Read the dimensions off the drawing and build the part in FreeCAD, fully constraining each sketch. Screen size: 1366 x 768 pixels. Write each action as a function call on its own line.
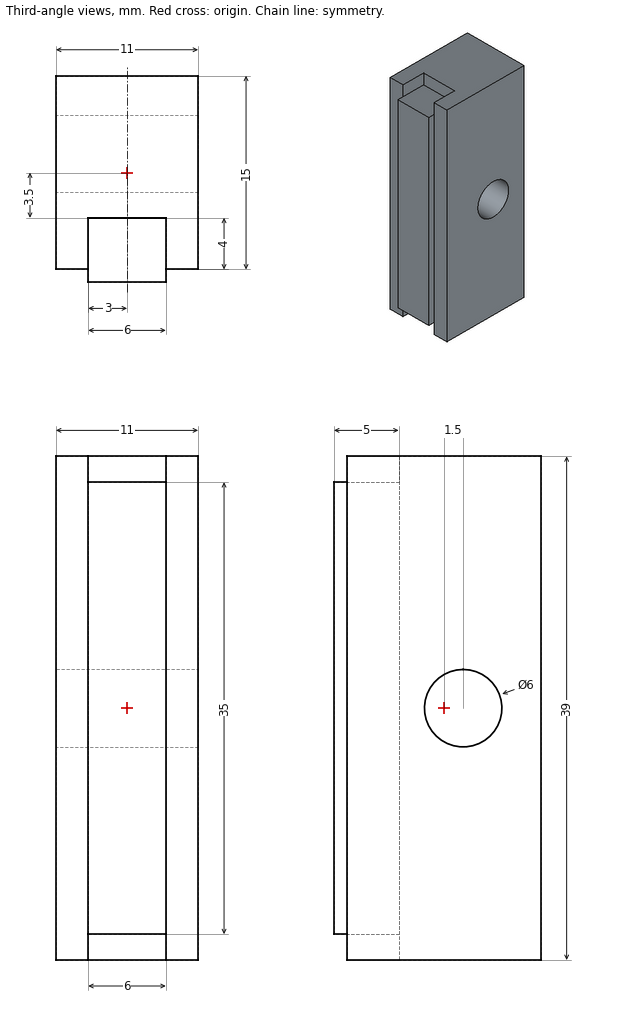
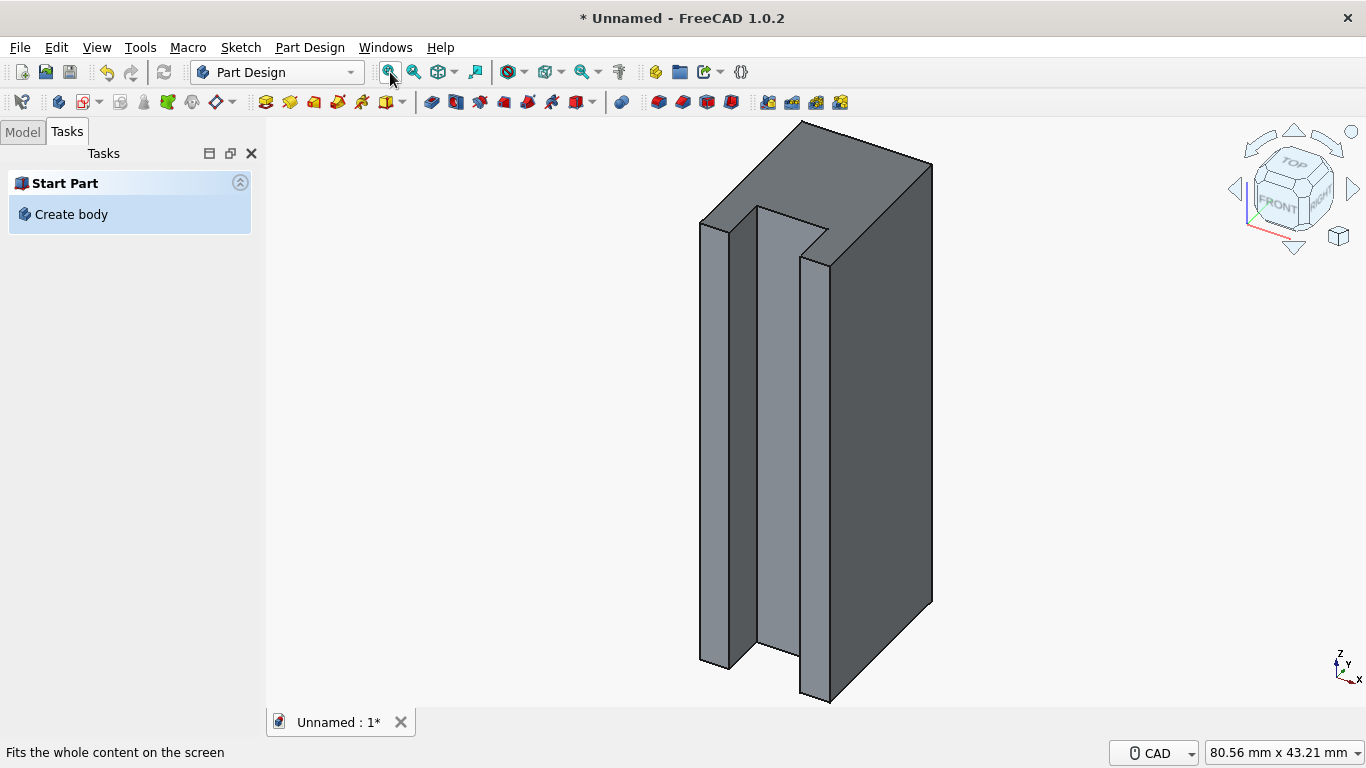
key(6)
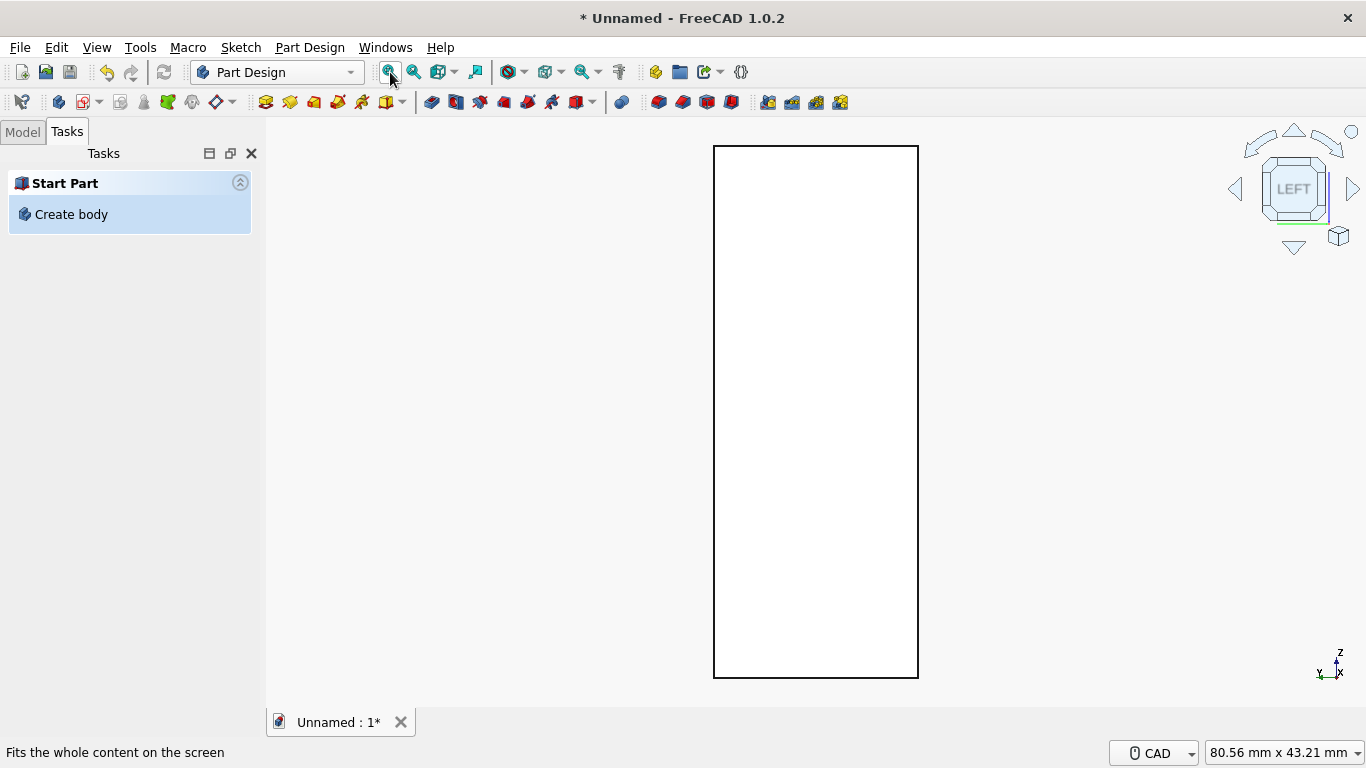
click(816, 259)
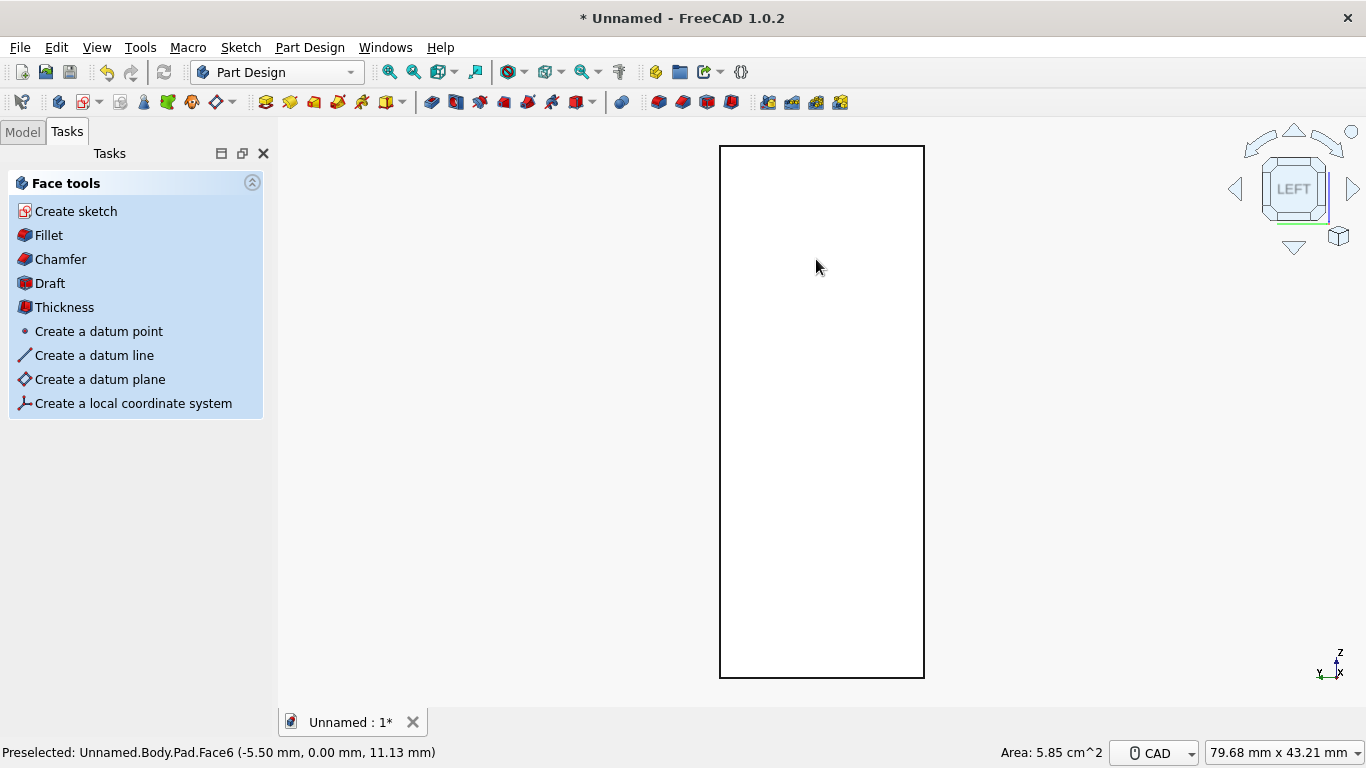
click(84, 102)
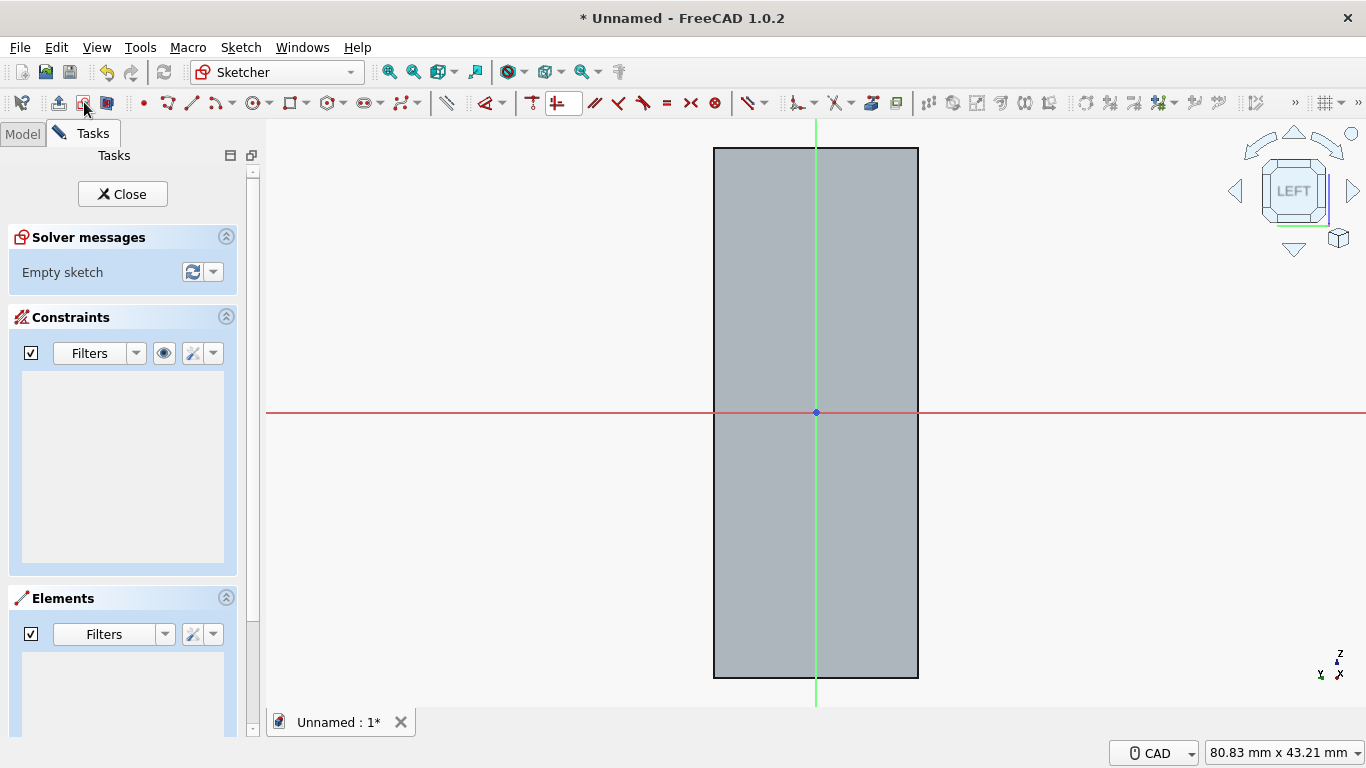
scroll(808, 413, up, 8)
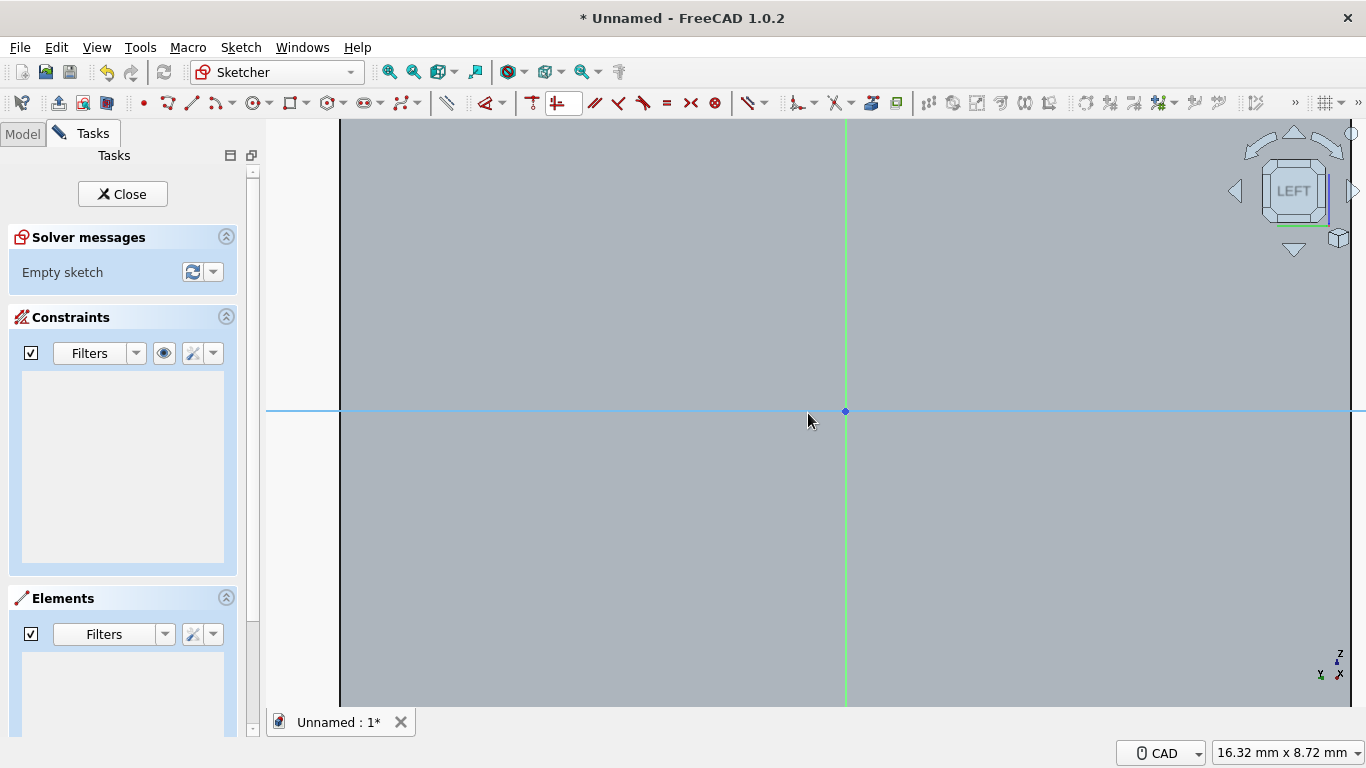
click(254, 104)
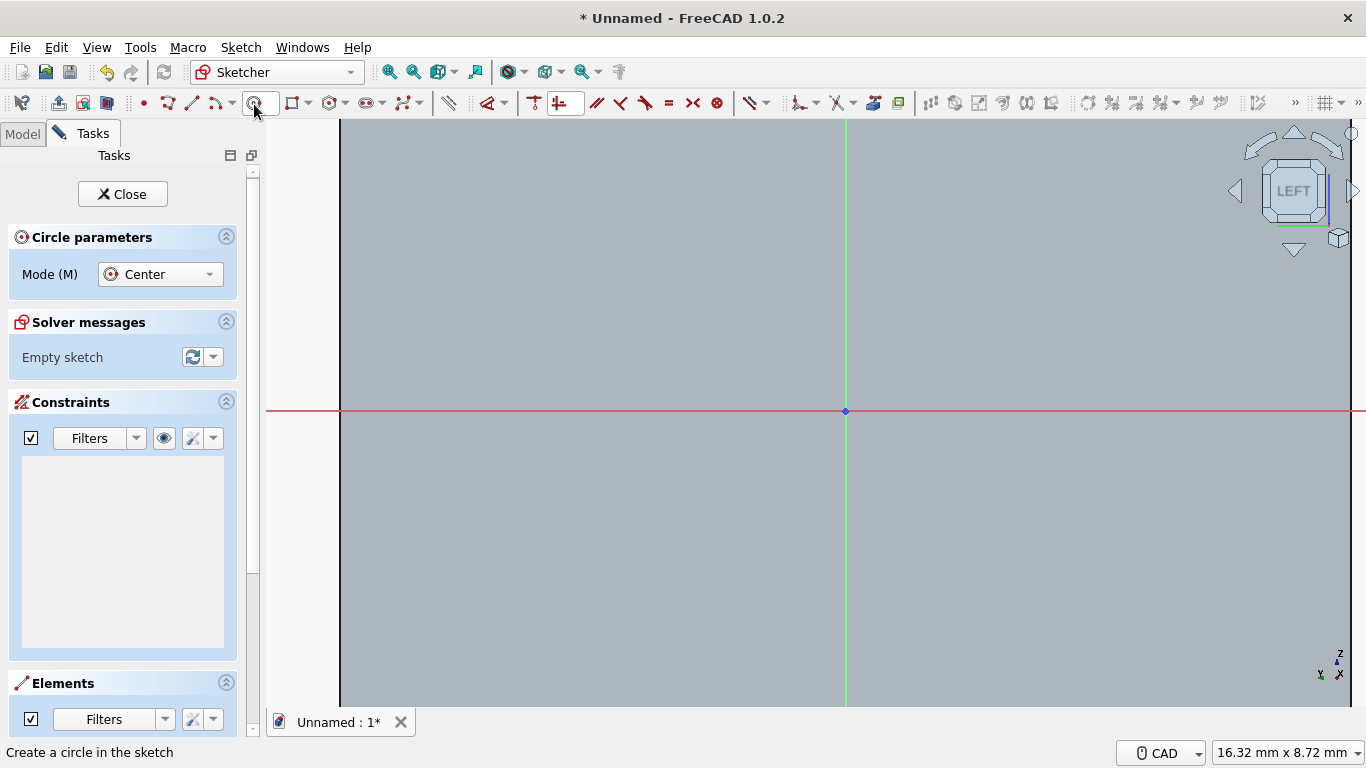
click(745, 411)
click(888, 268)
key(Escape)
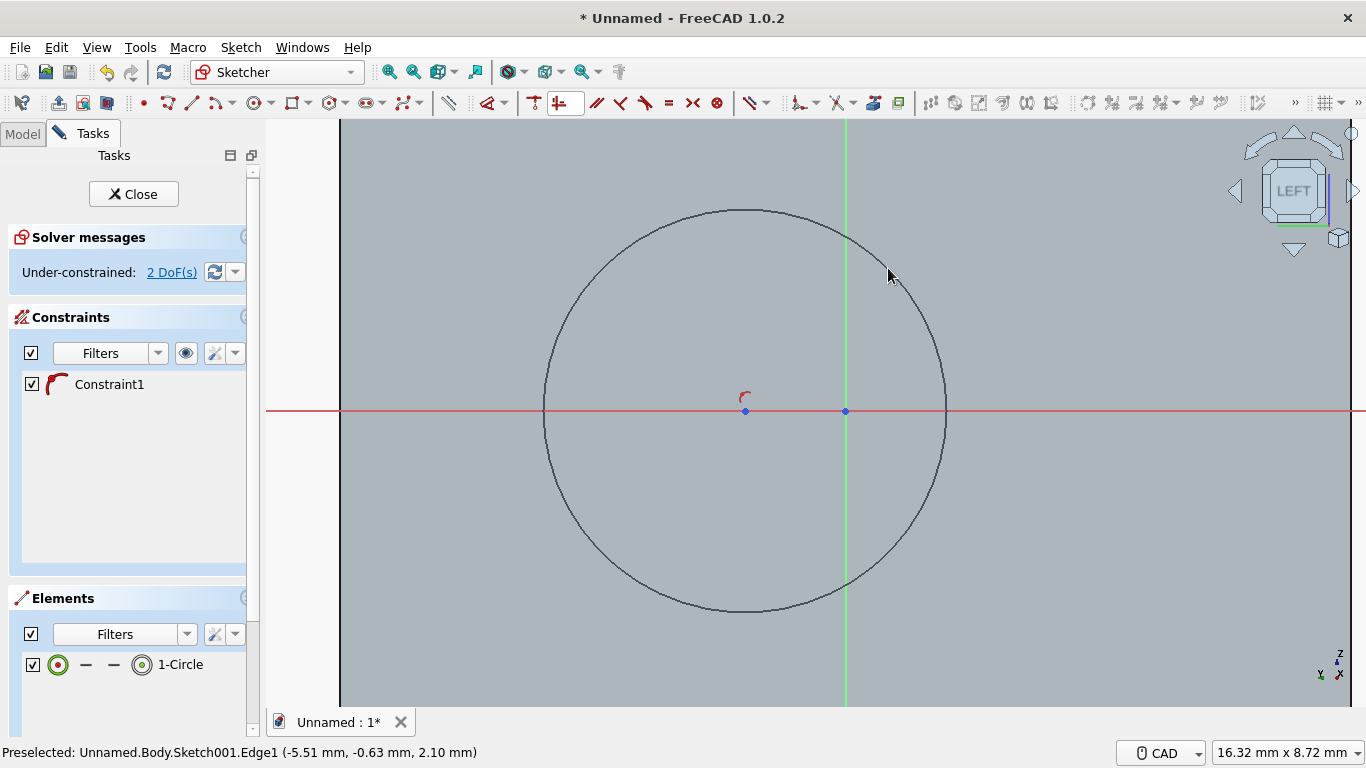
click(488, 104)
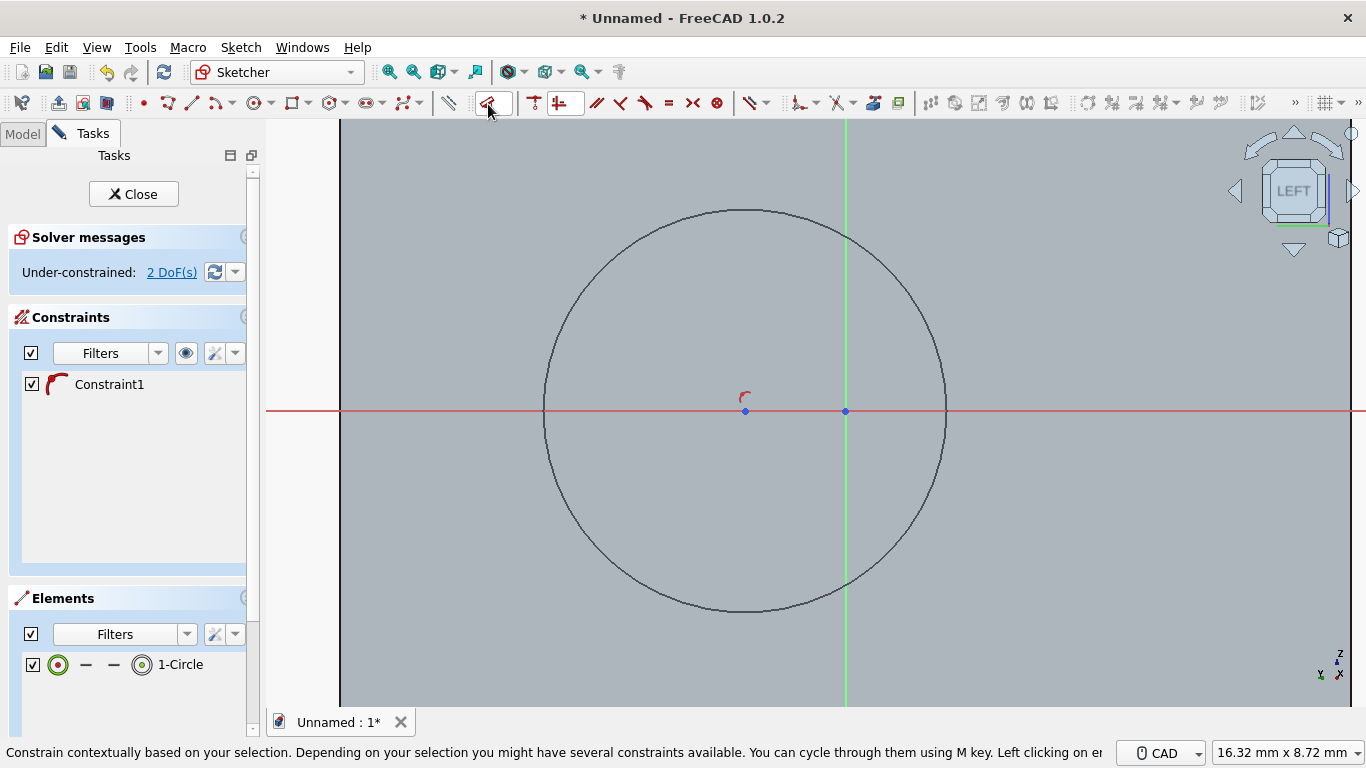
click(887, 268)
click(910, 245)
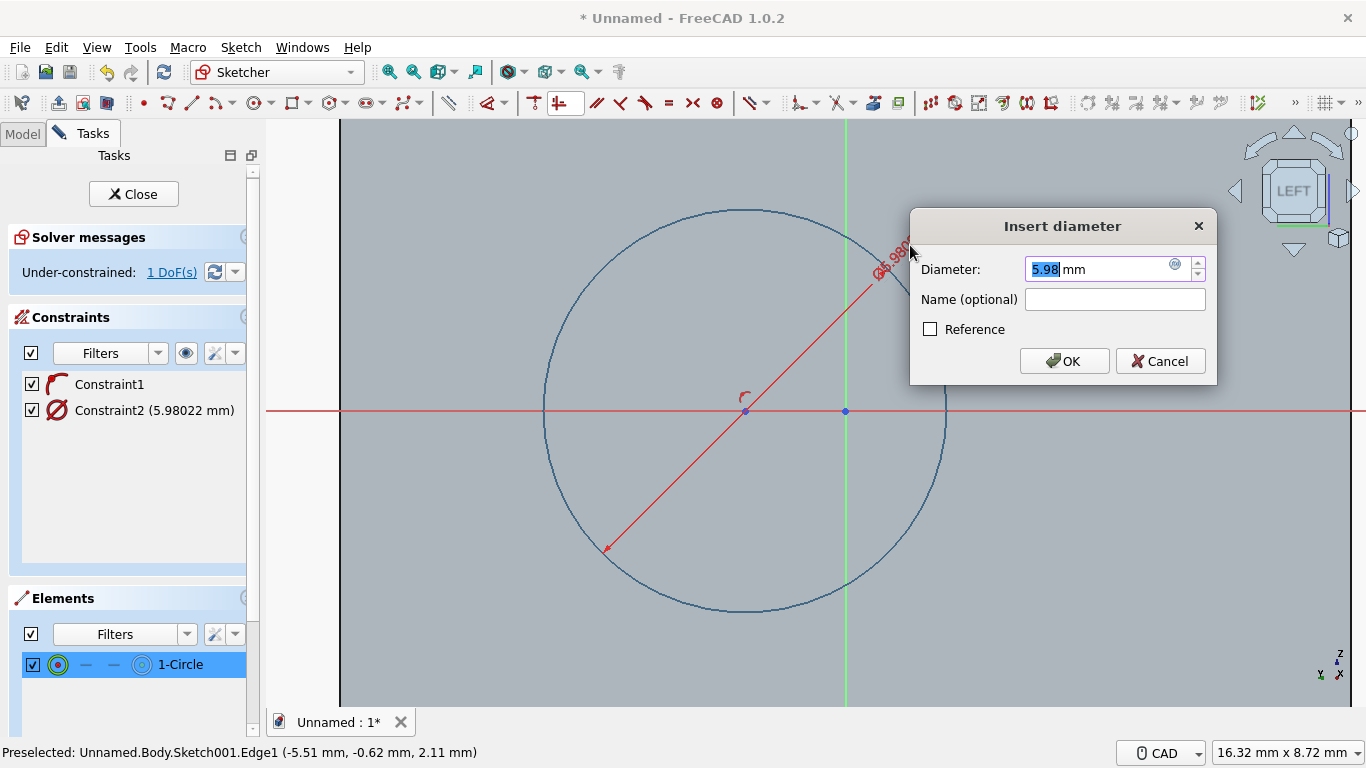
text(6)
key(Return)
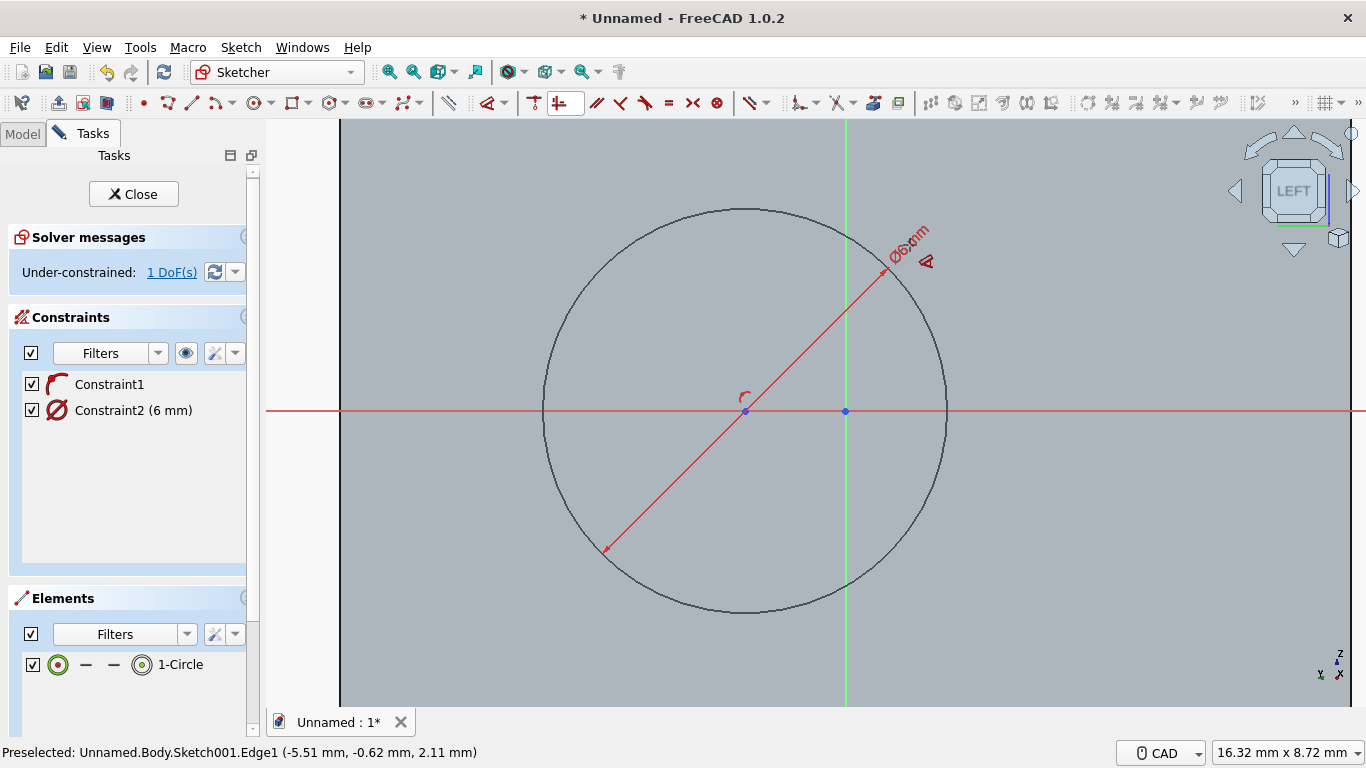
click(745, 411)
click(795, 445)